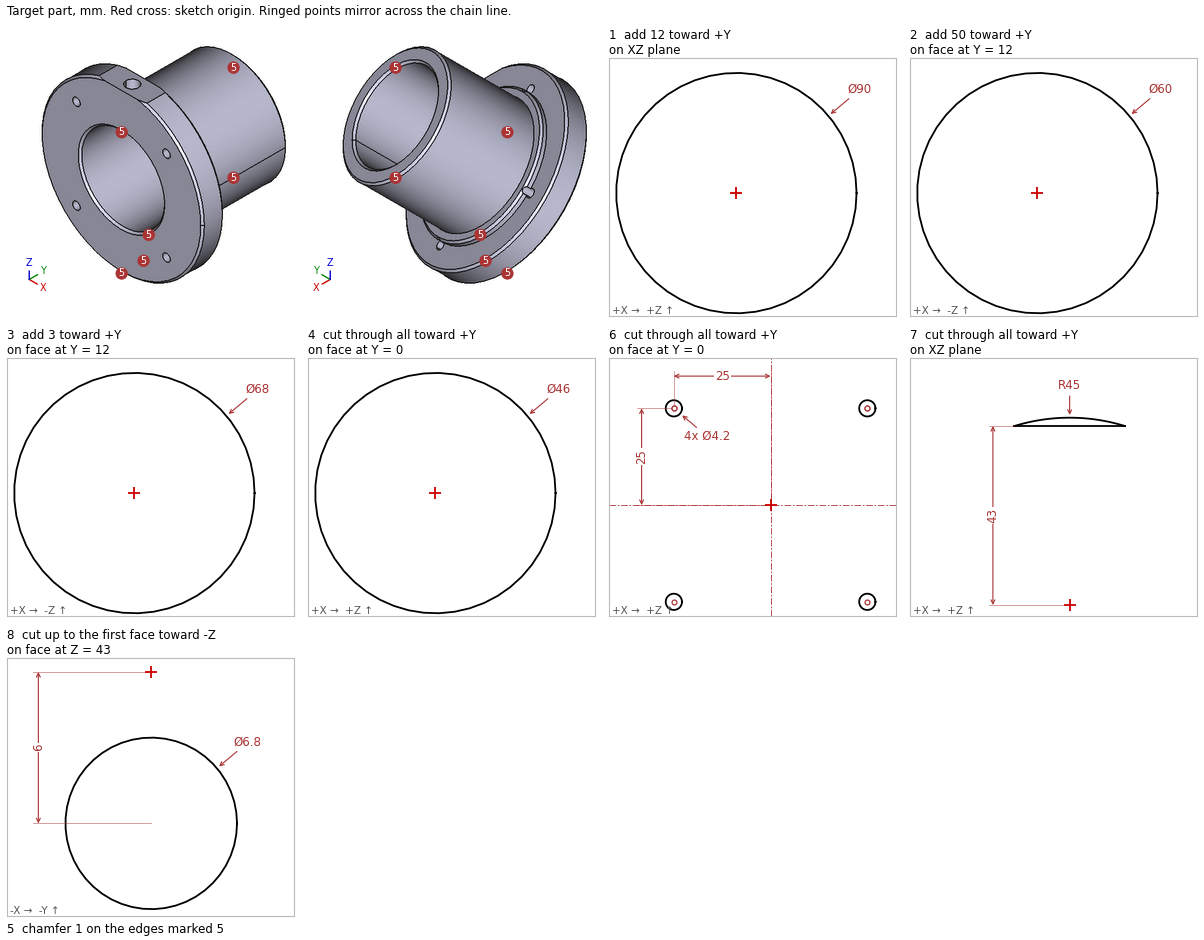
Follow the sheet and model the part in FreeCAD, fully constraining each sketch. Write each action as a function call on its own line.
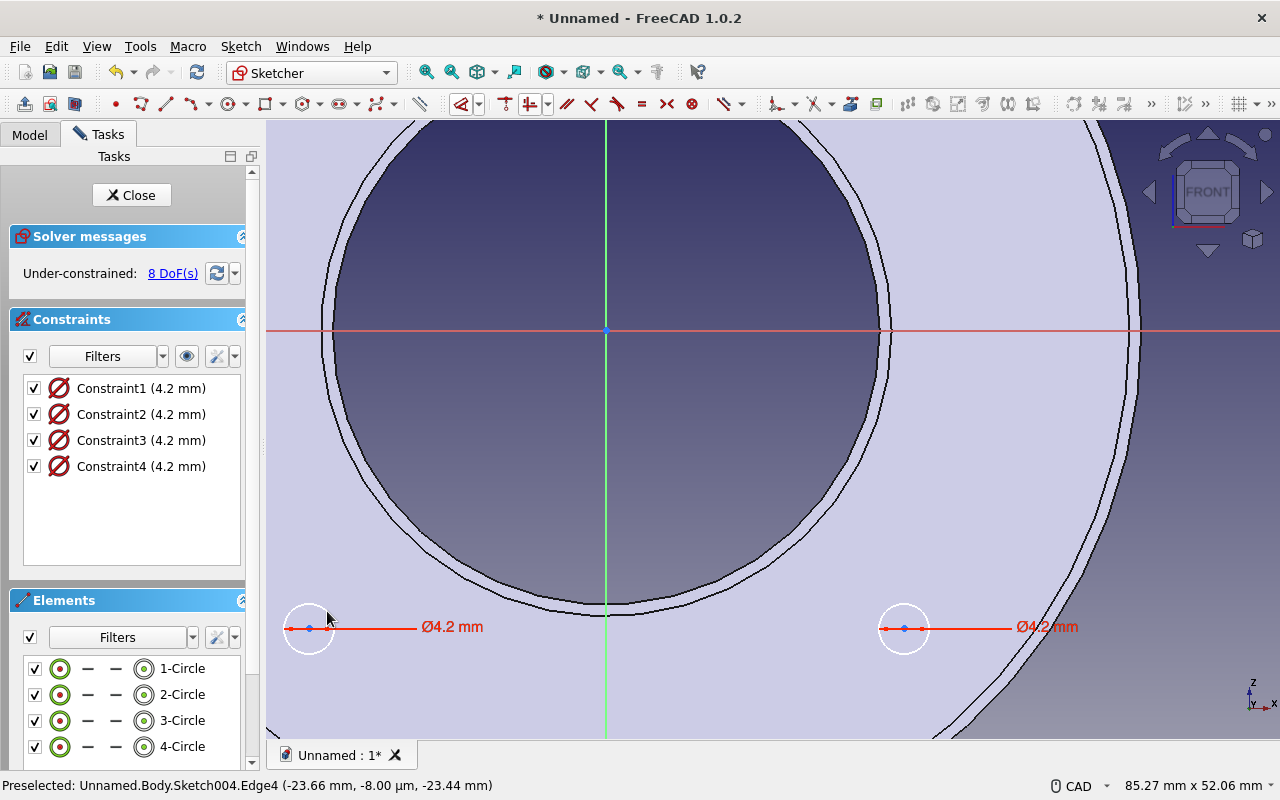
scroll(904, 630, down, 2)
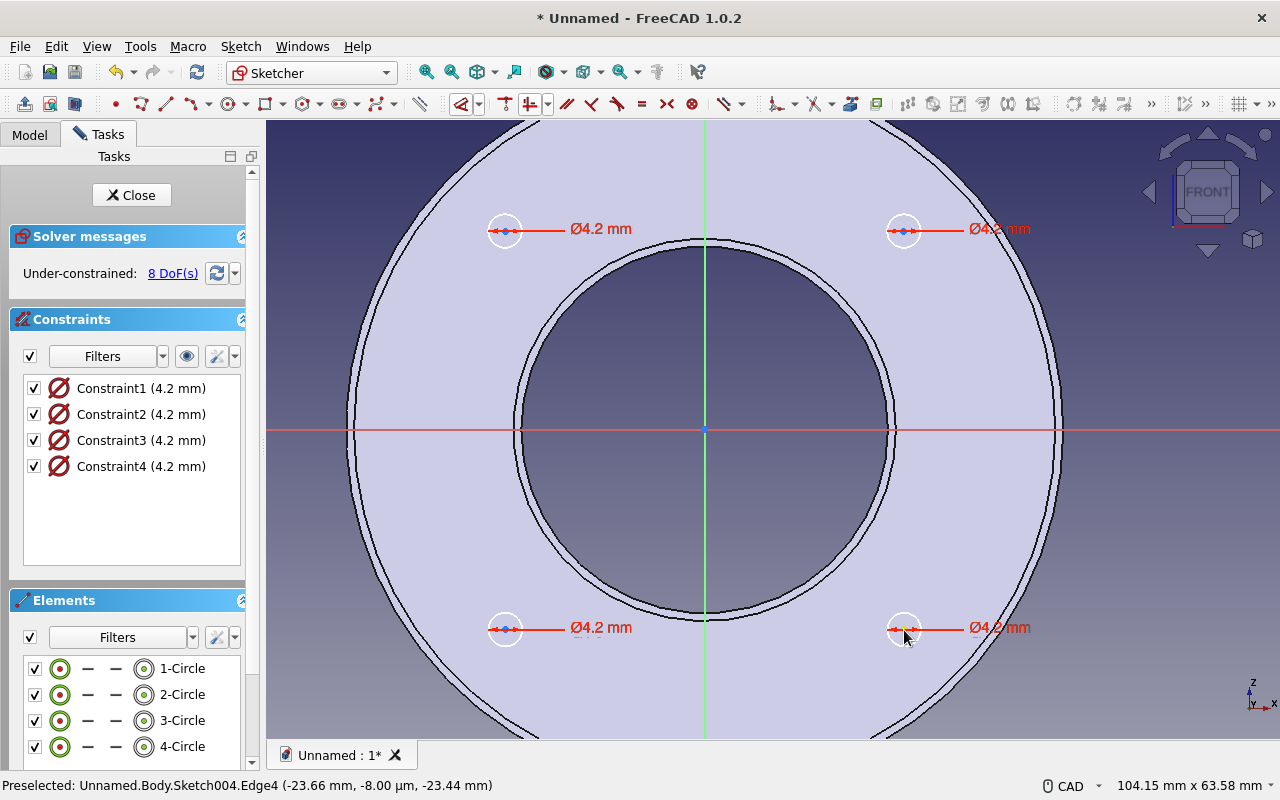
click(505, 231)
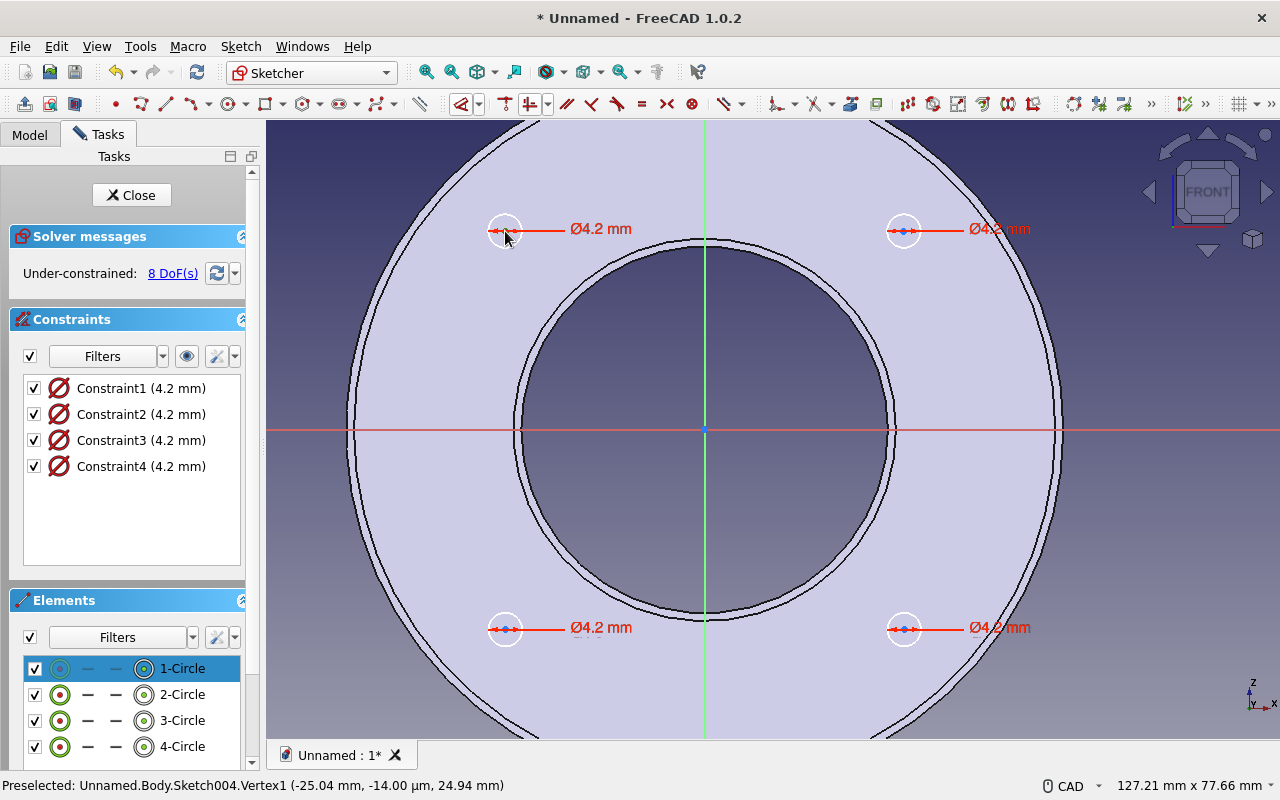
click(904, 231)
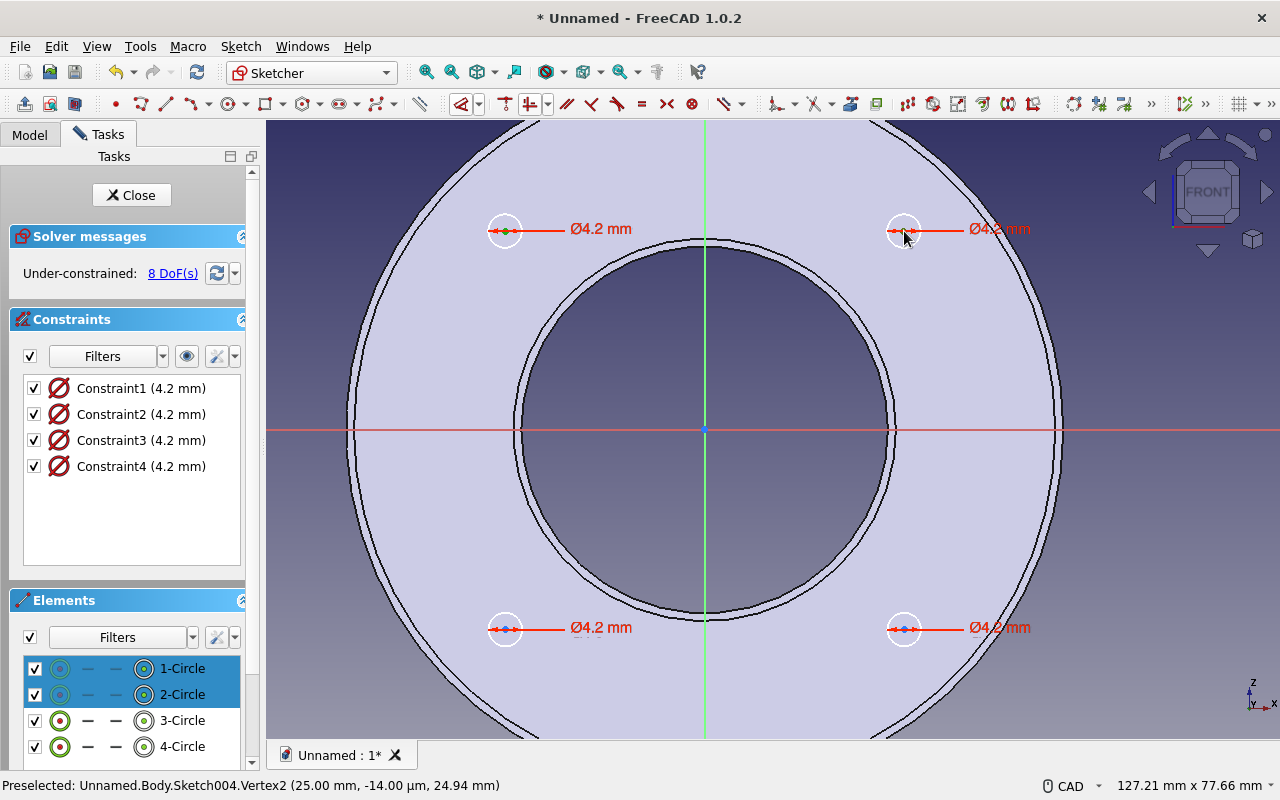
click(705, 671)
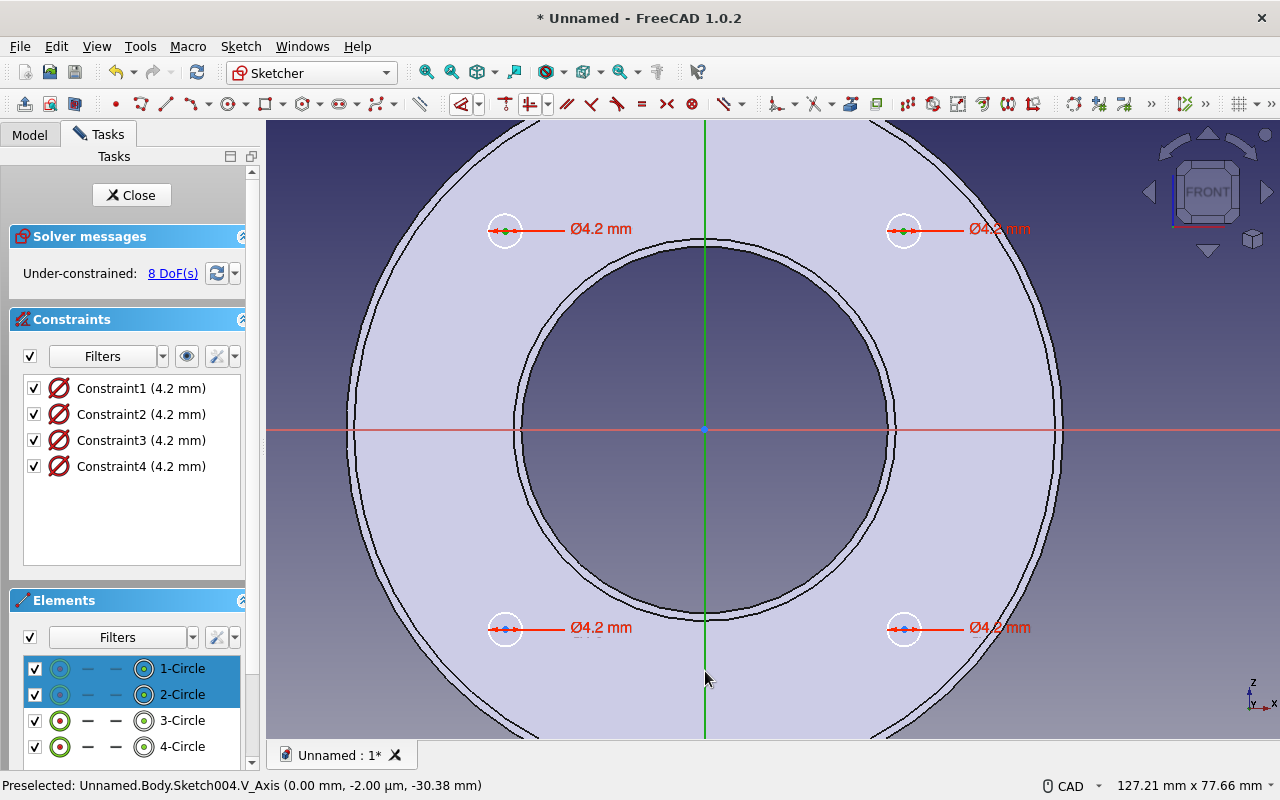
click(667, 104)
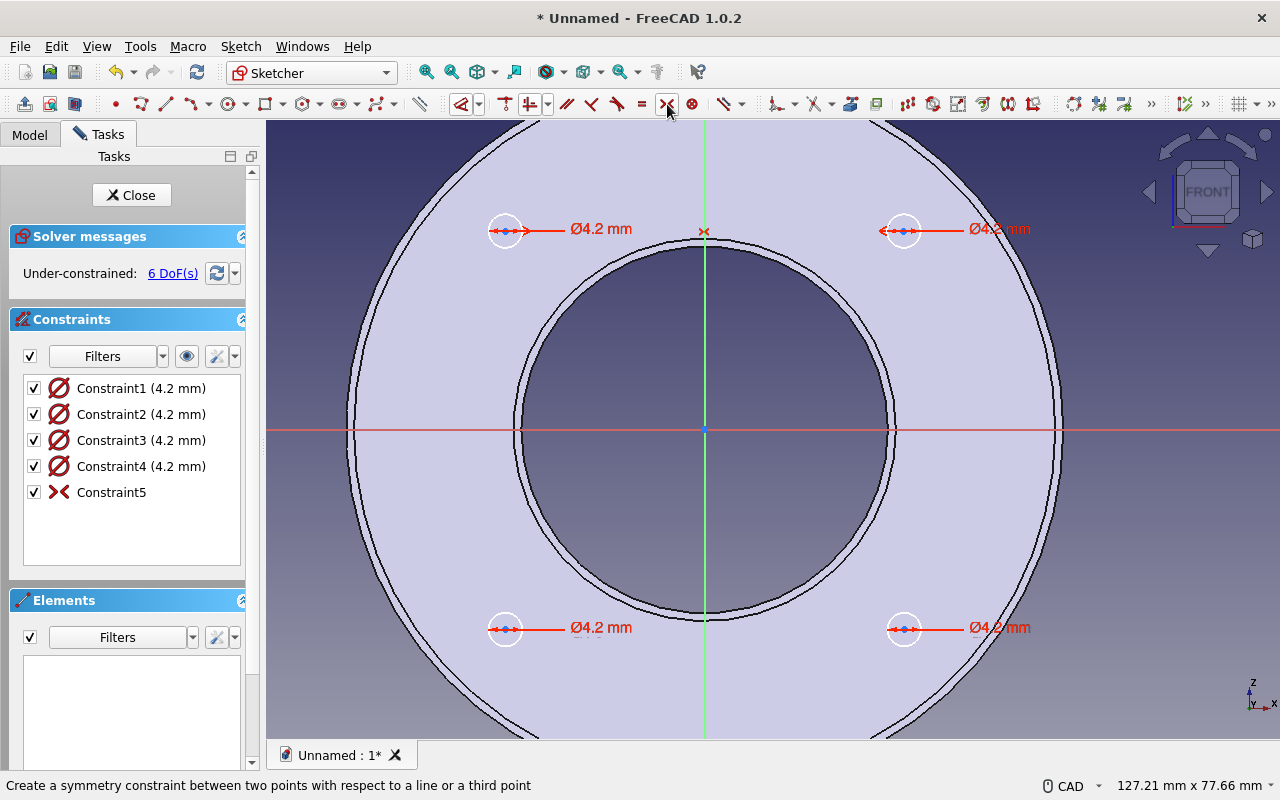
click(904, 231)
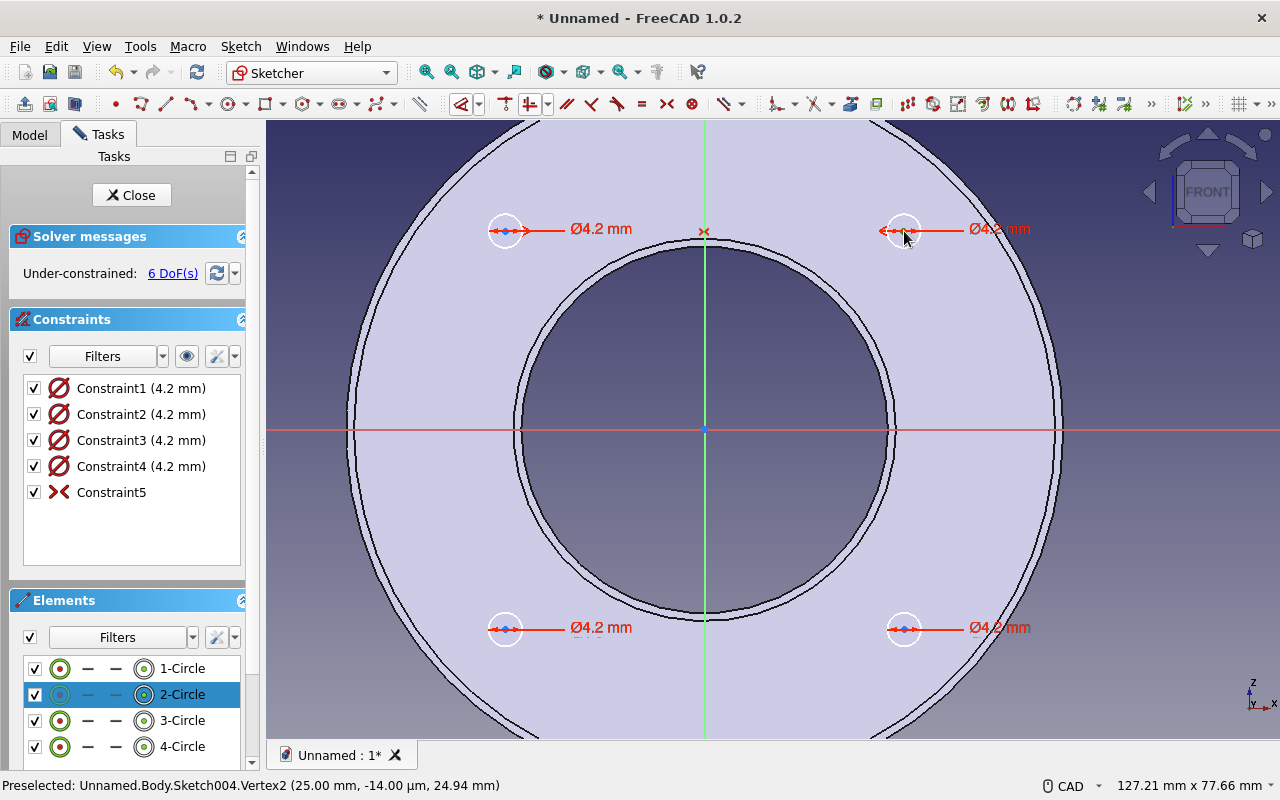
click(904, 630)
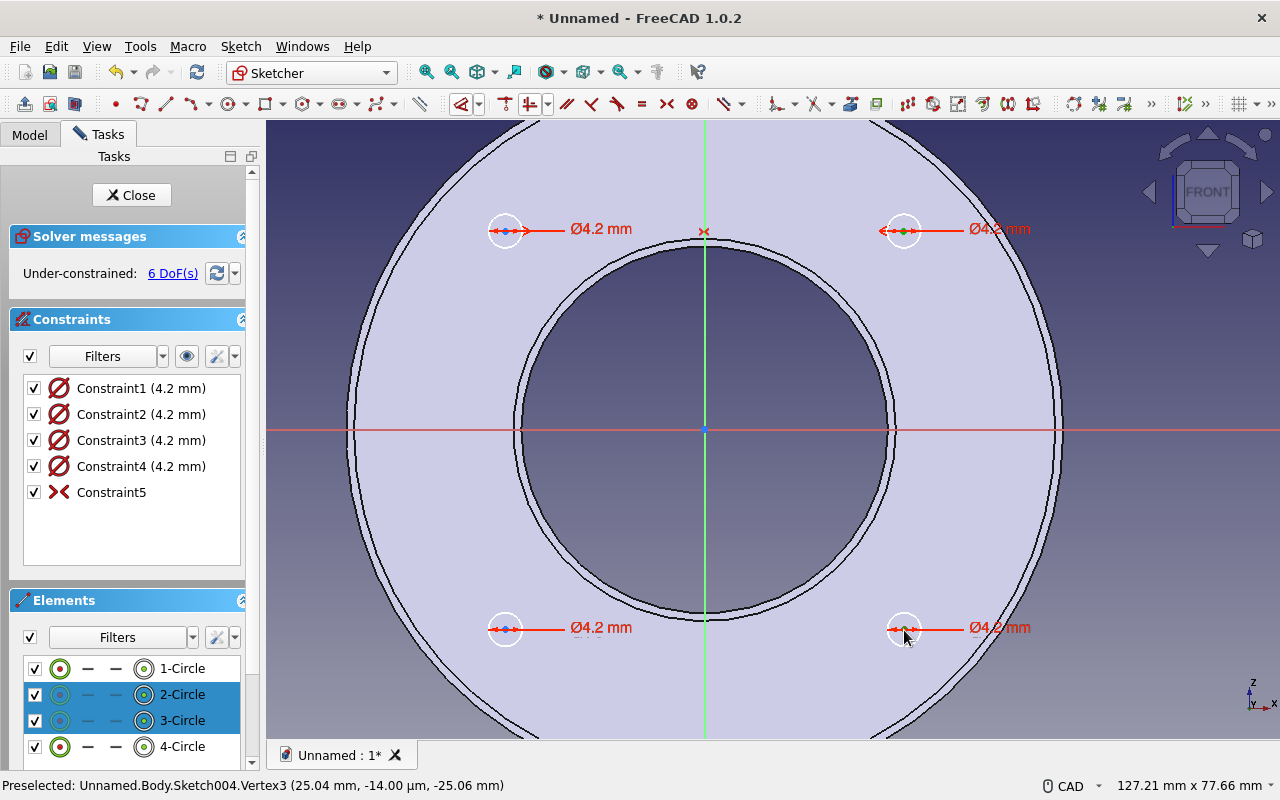
click(353, 430)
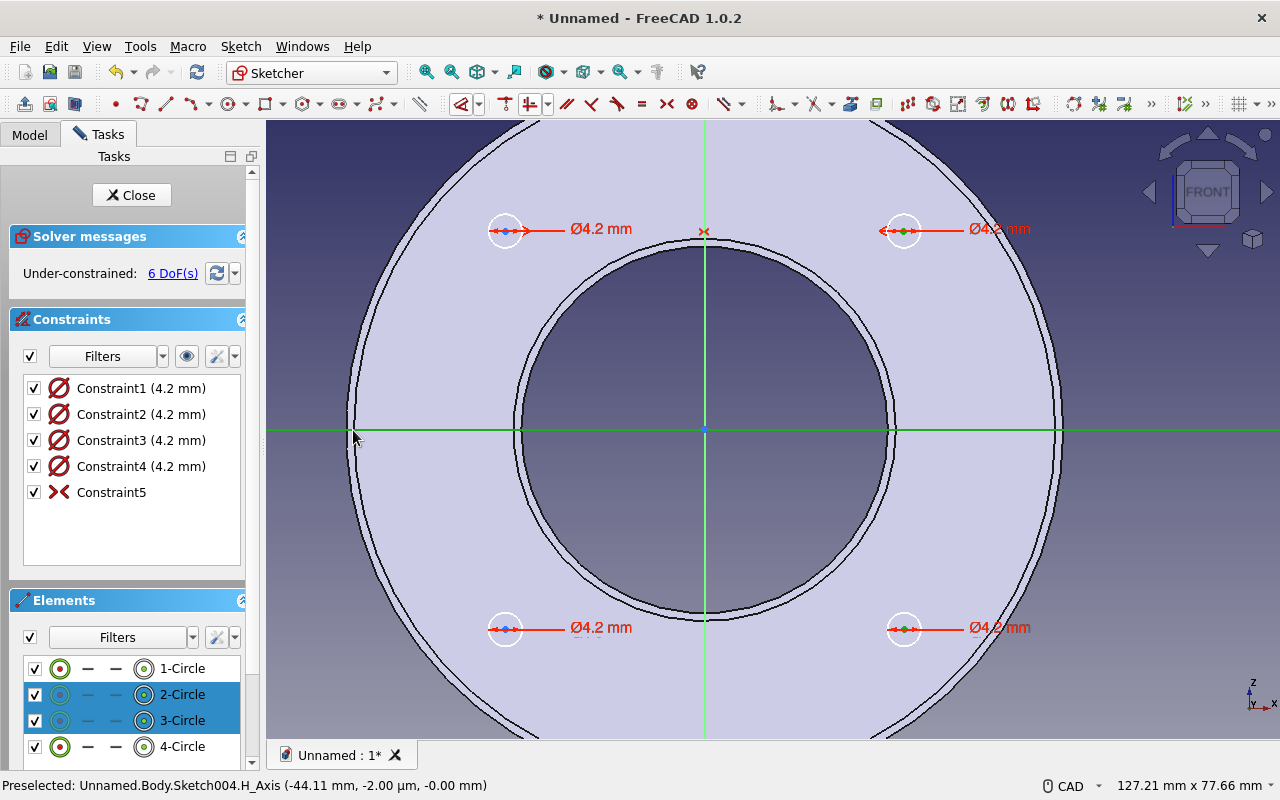
click(667, 104)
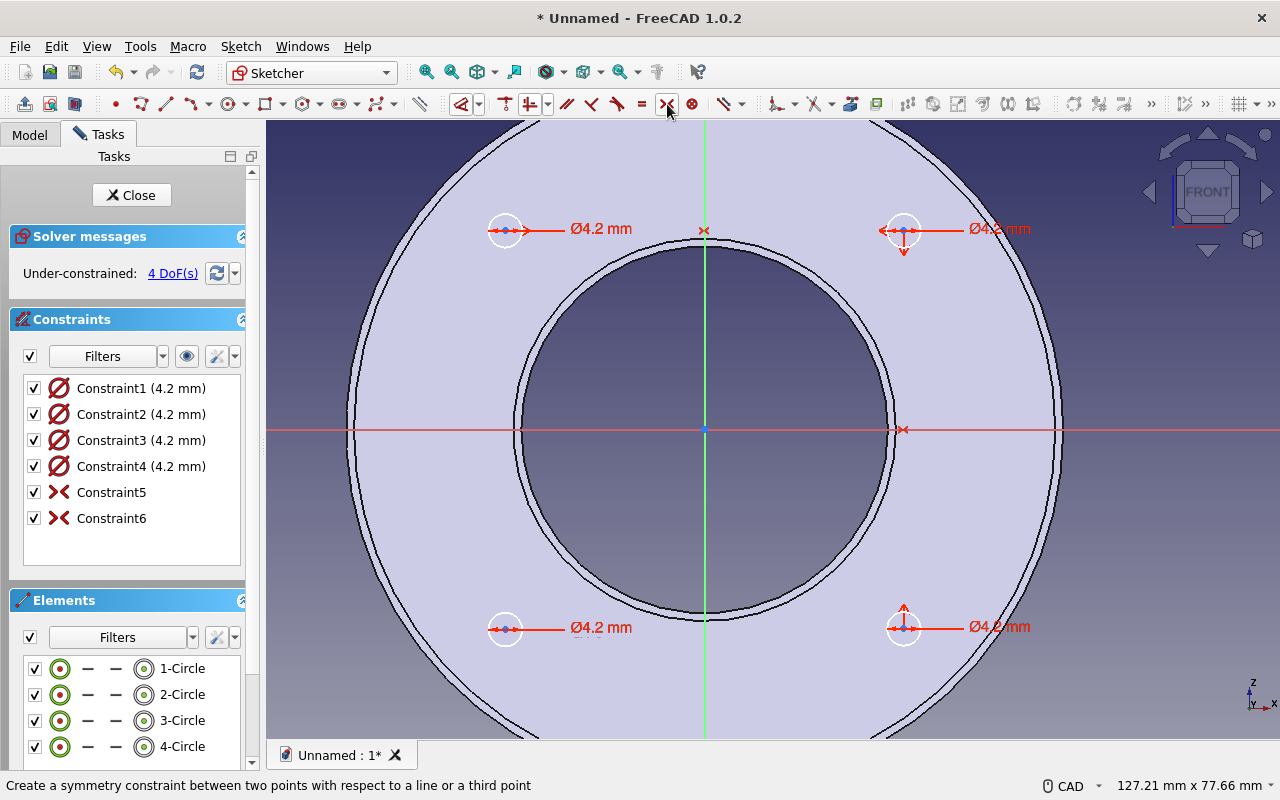
click(505, 231)